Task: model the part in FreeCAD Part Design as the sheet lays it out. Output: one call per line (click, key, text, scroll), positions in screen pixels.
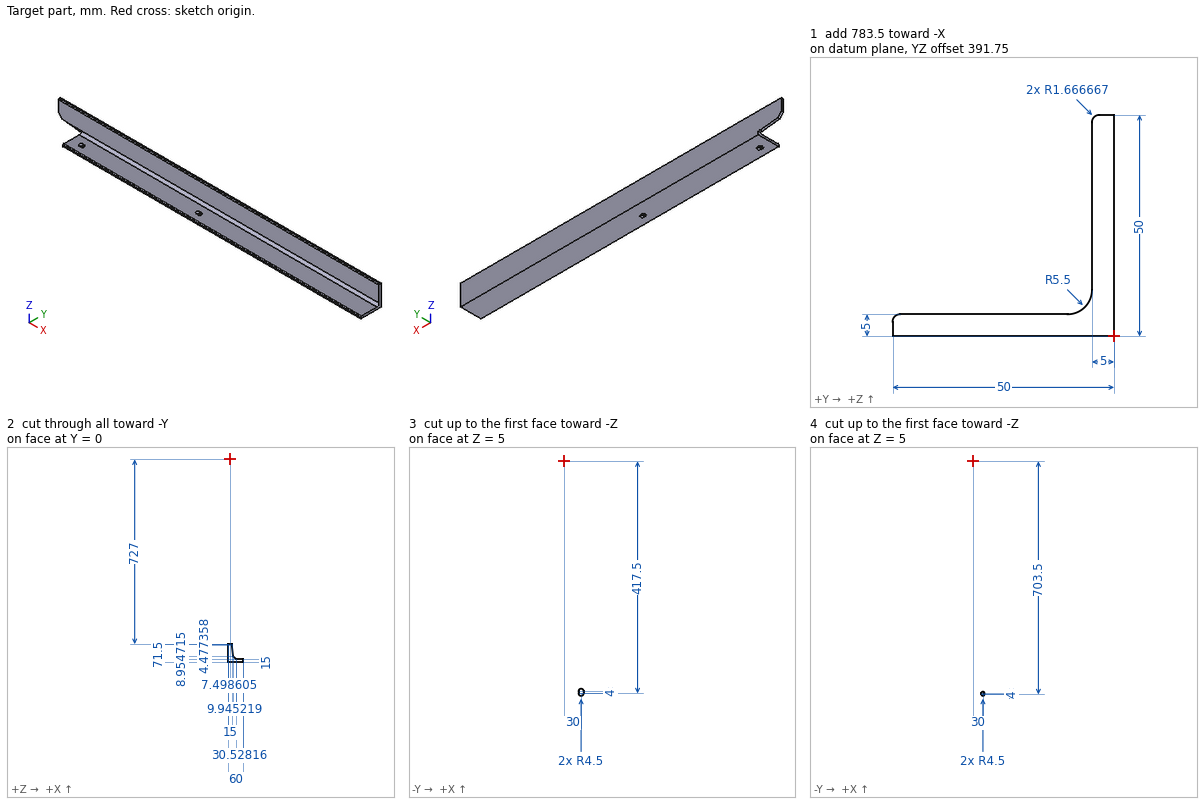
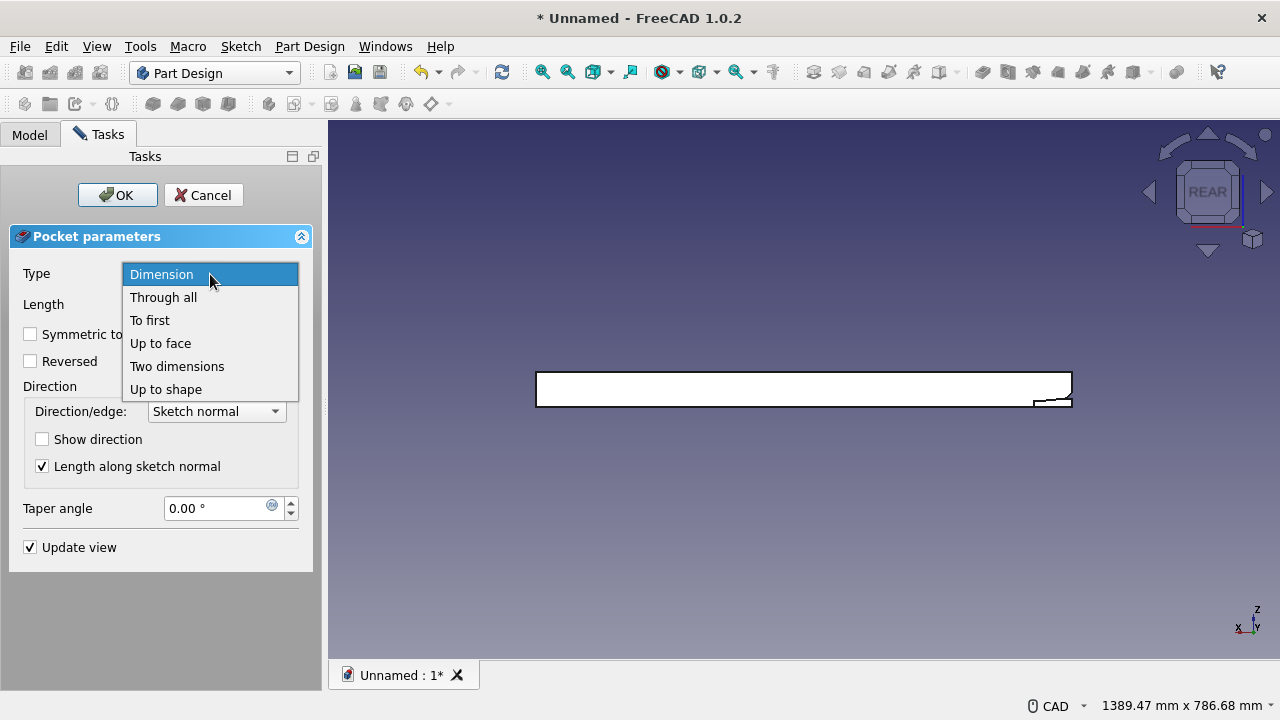
click(208, 298)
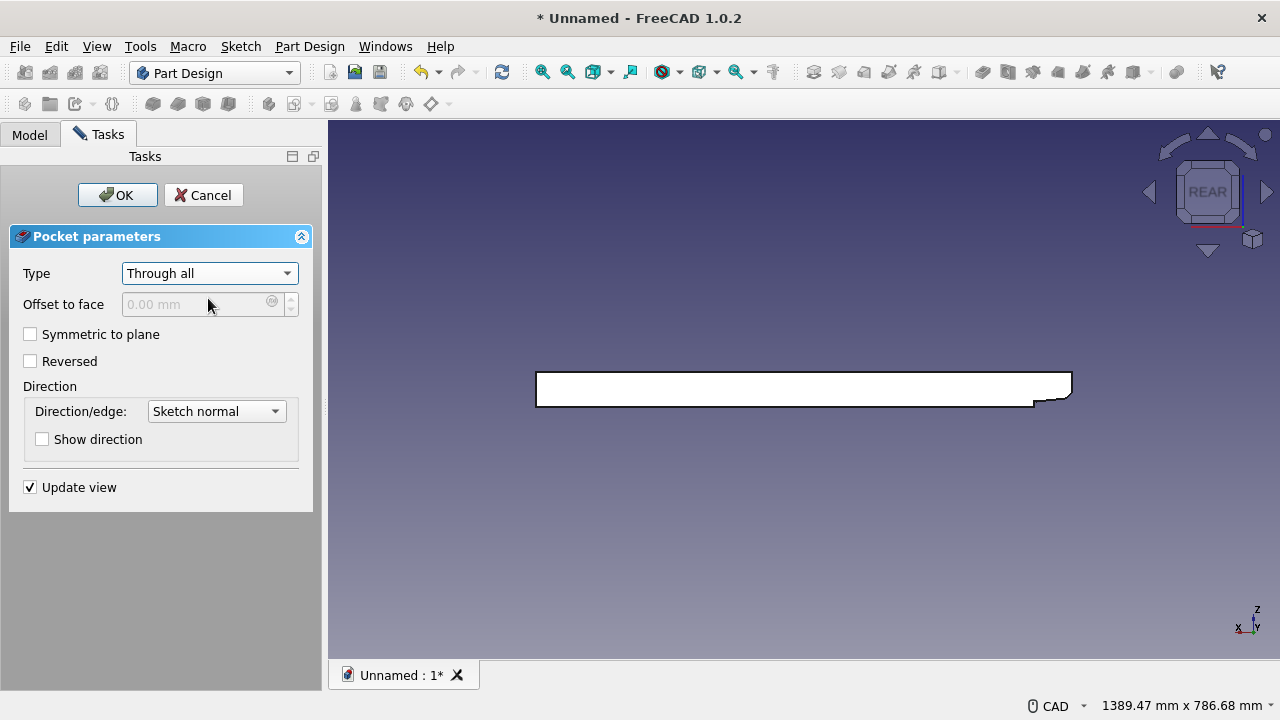
click(118, 195)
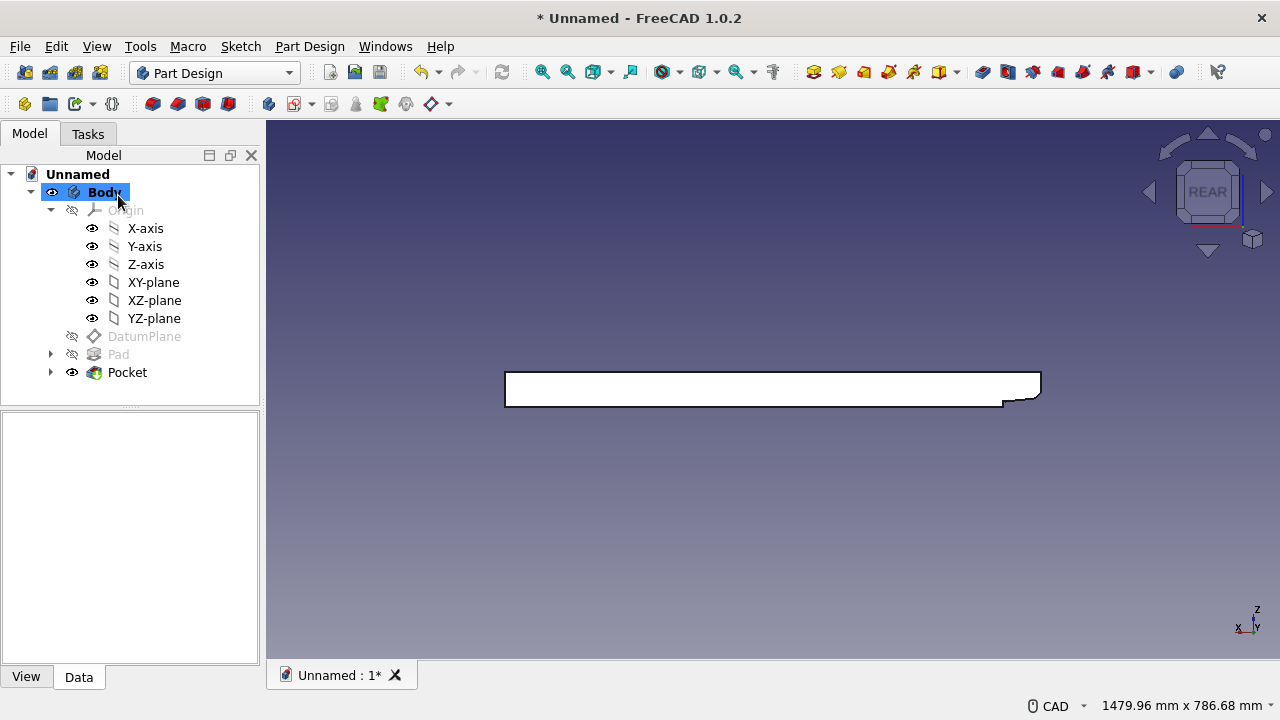
key(0)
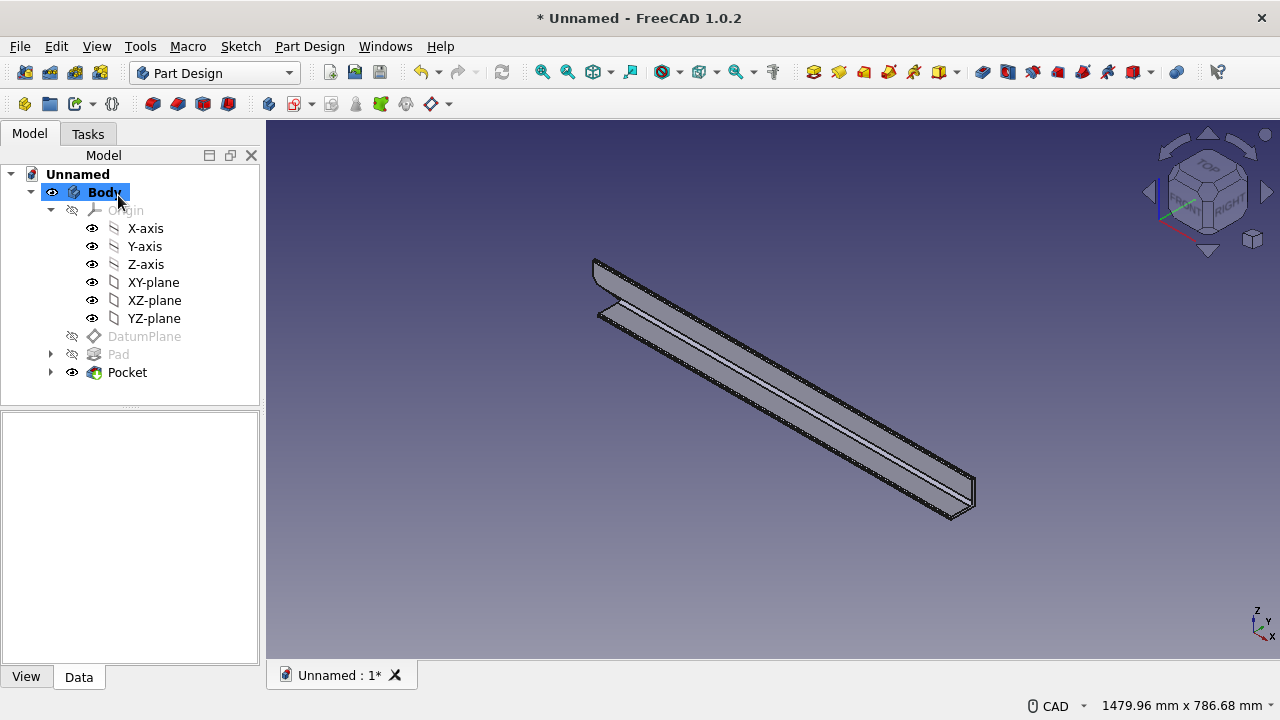
click(785, 409)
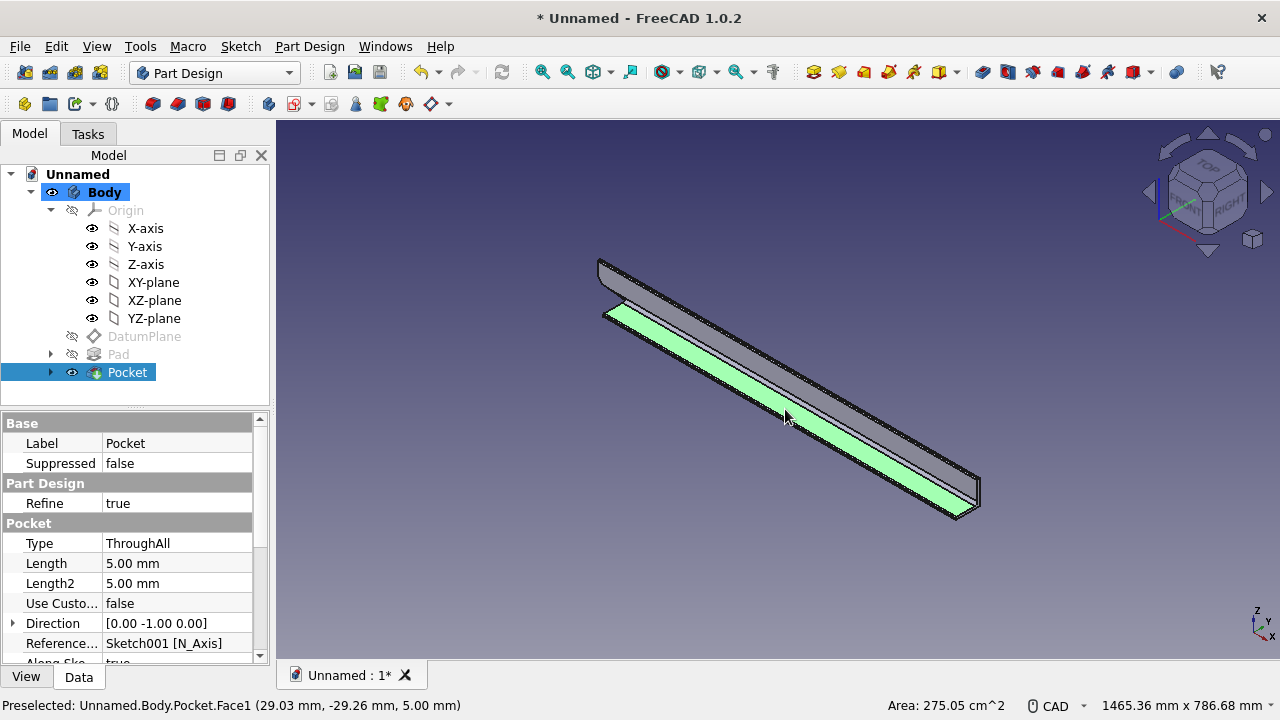
click(294, 104)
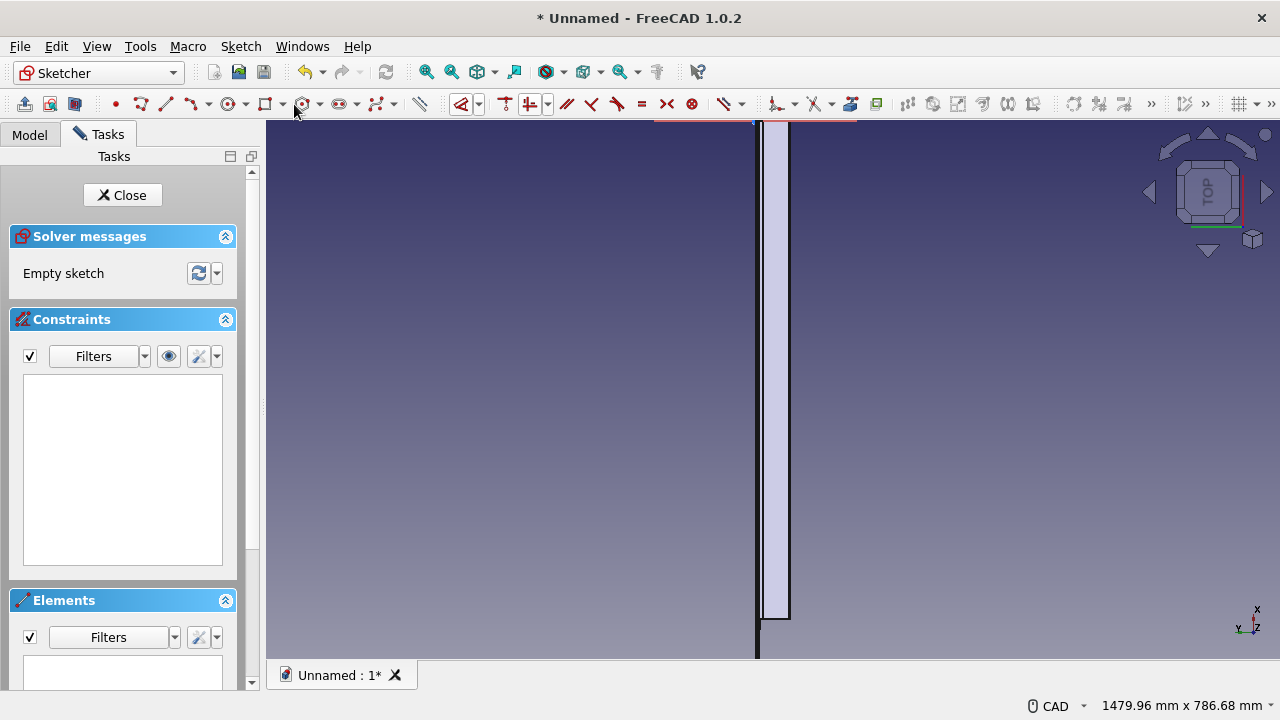
click(75, 104)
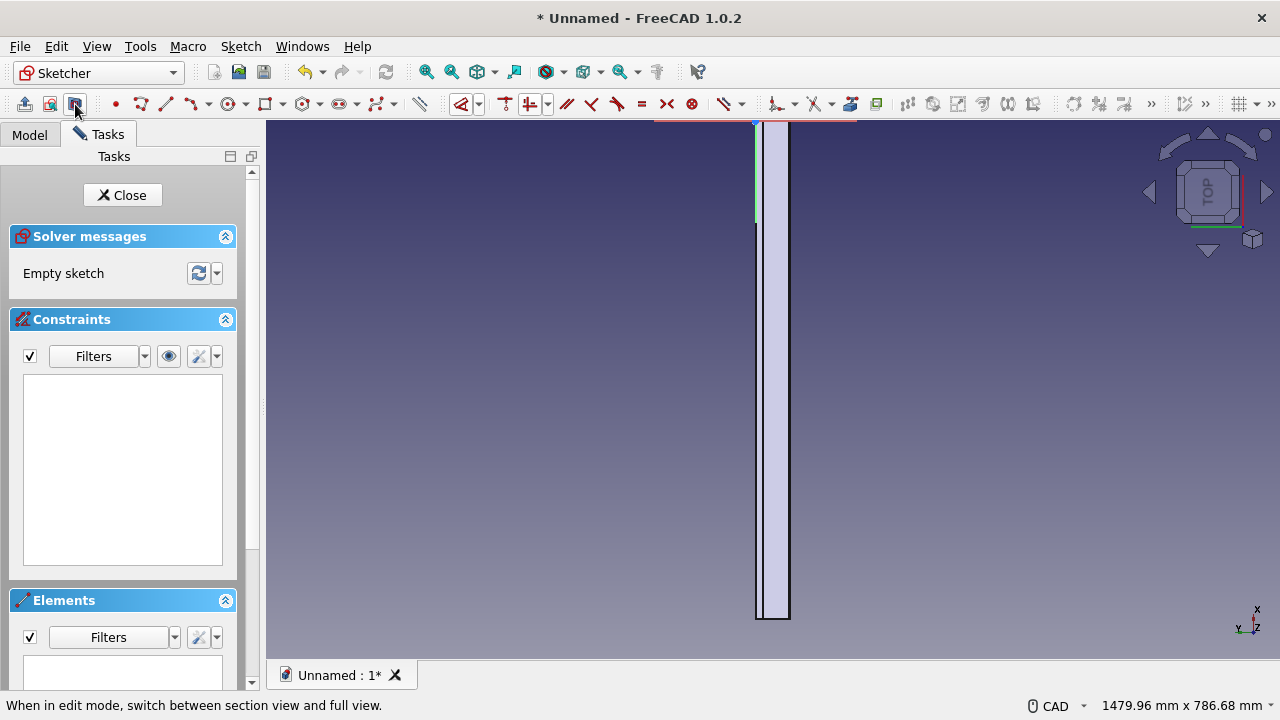
scroll(780, 407, up, 15)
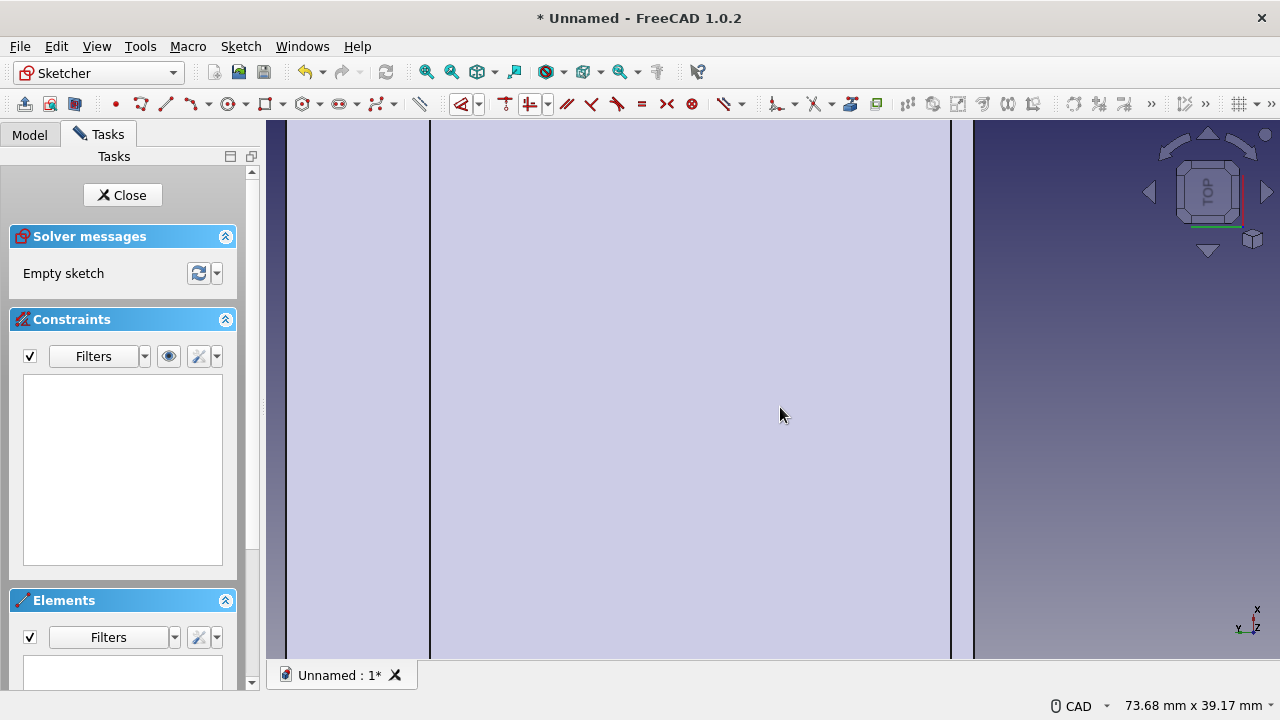
scroll(691, 351, up, 3)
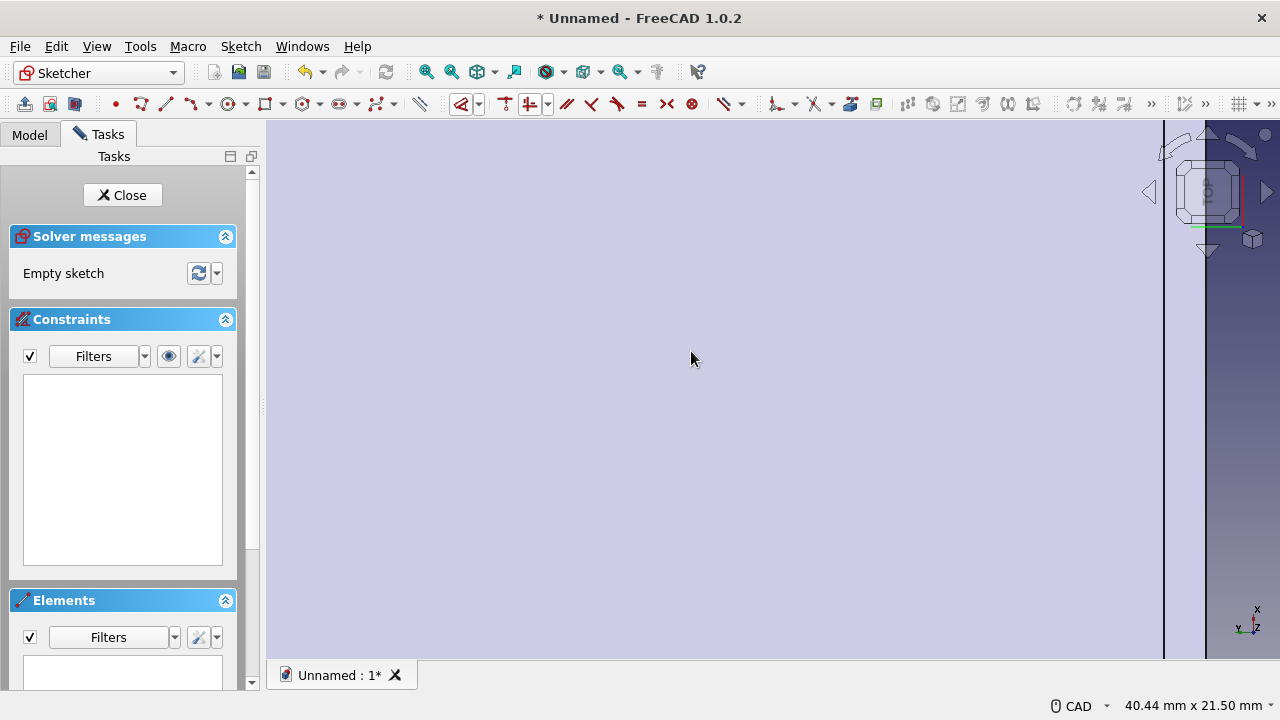
key(g)
key(s)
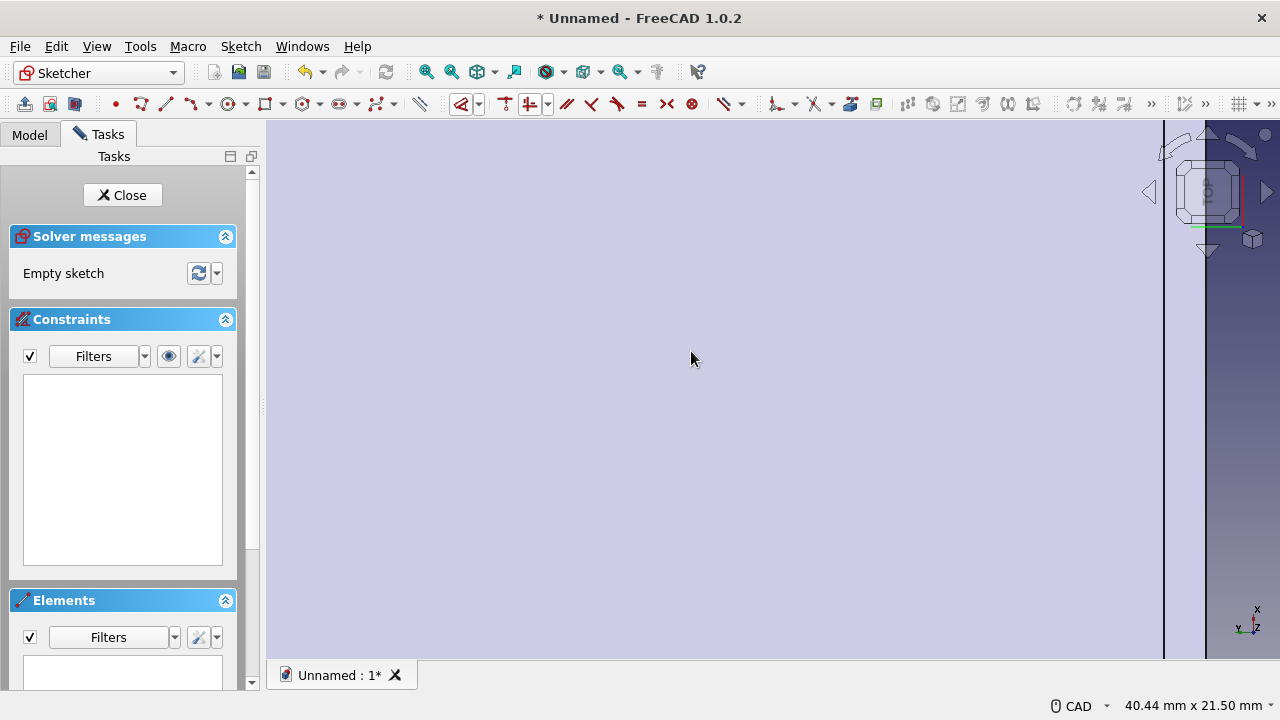
click(704, 439)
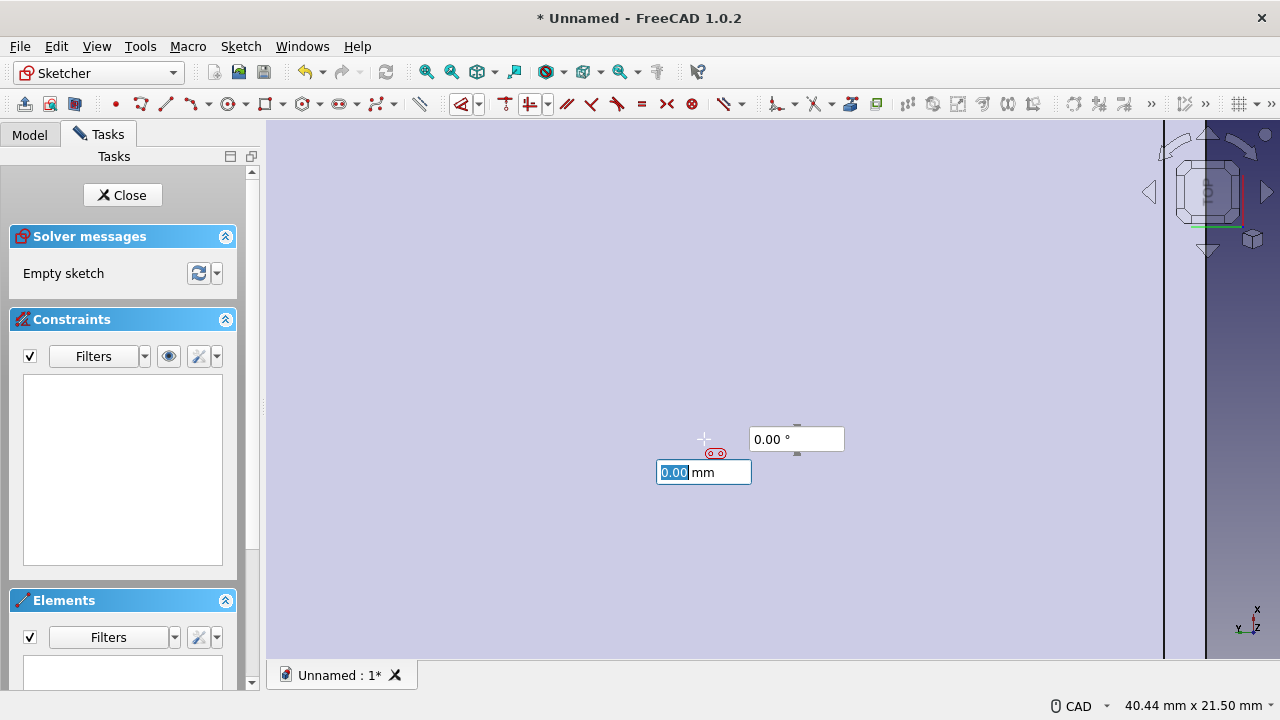
click(704, 339)